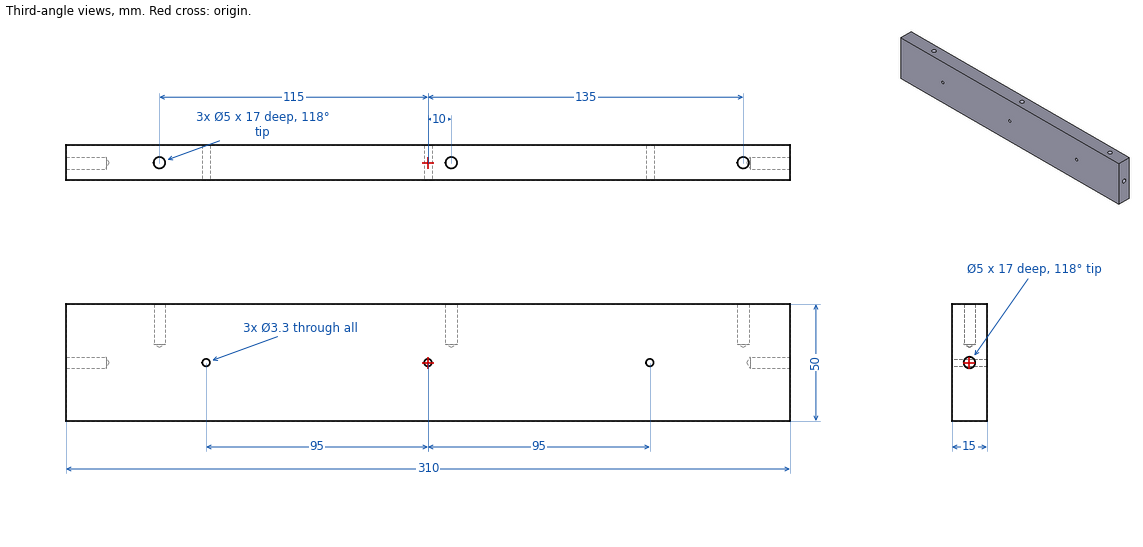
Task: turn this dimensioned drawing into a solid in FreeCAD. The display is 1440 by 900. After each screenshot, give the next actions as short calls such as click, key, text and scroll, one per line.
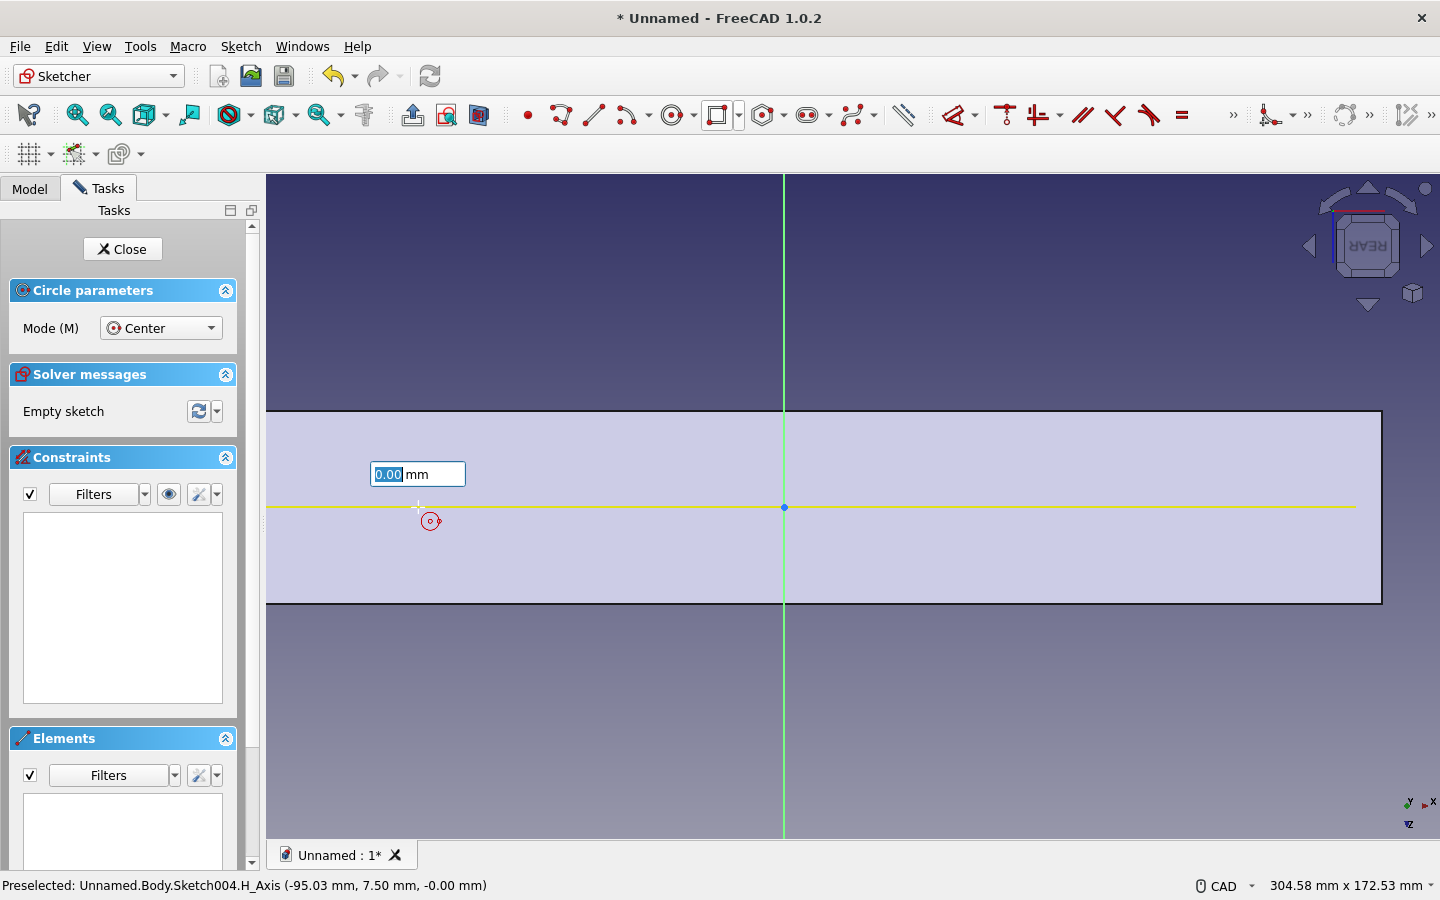
scroll(416, 513, up, 5)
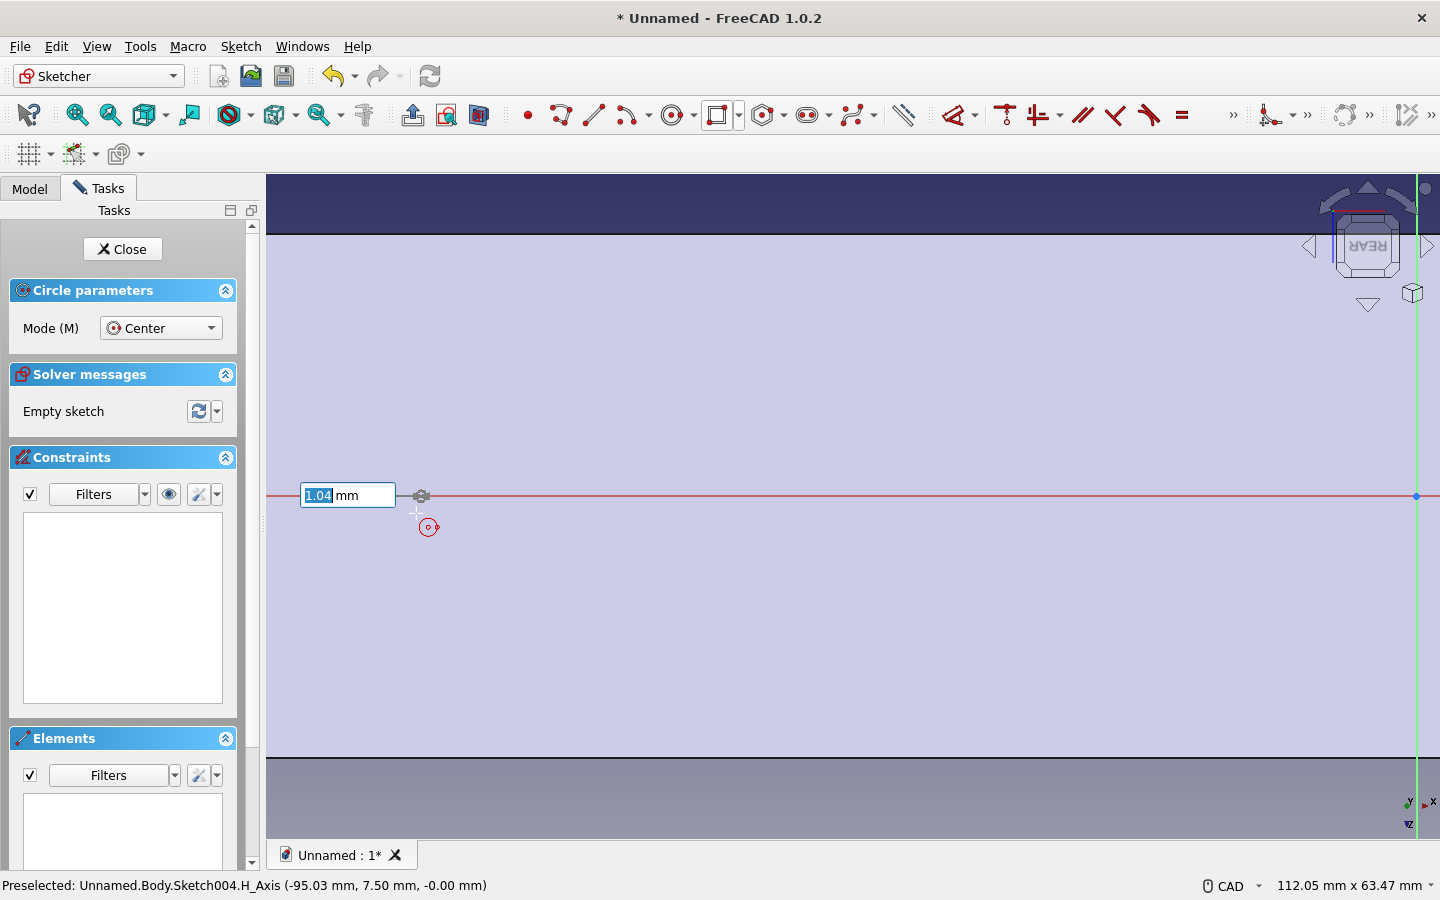
click(416, 513)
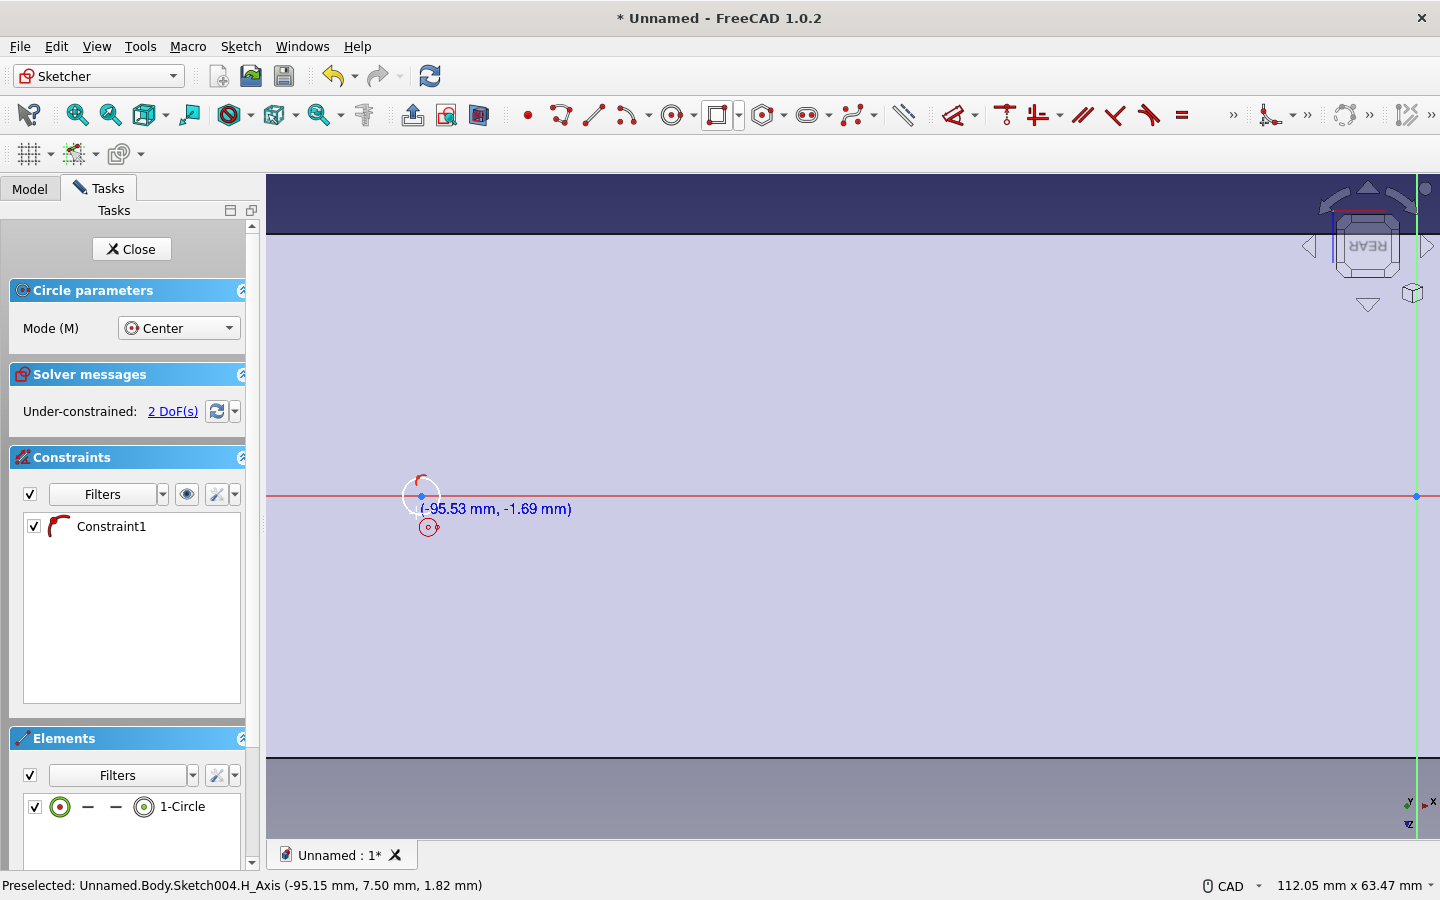
scroll(416, 512, down, 5)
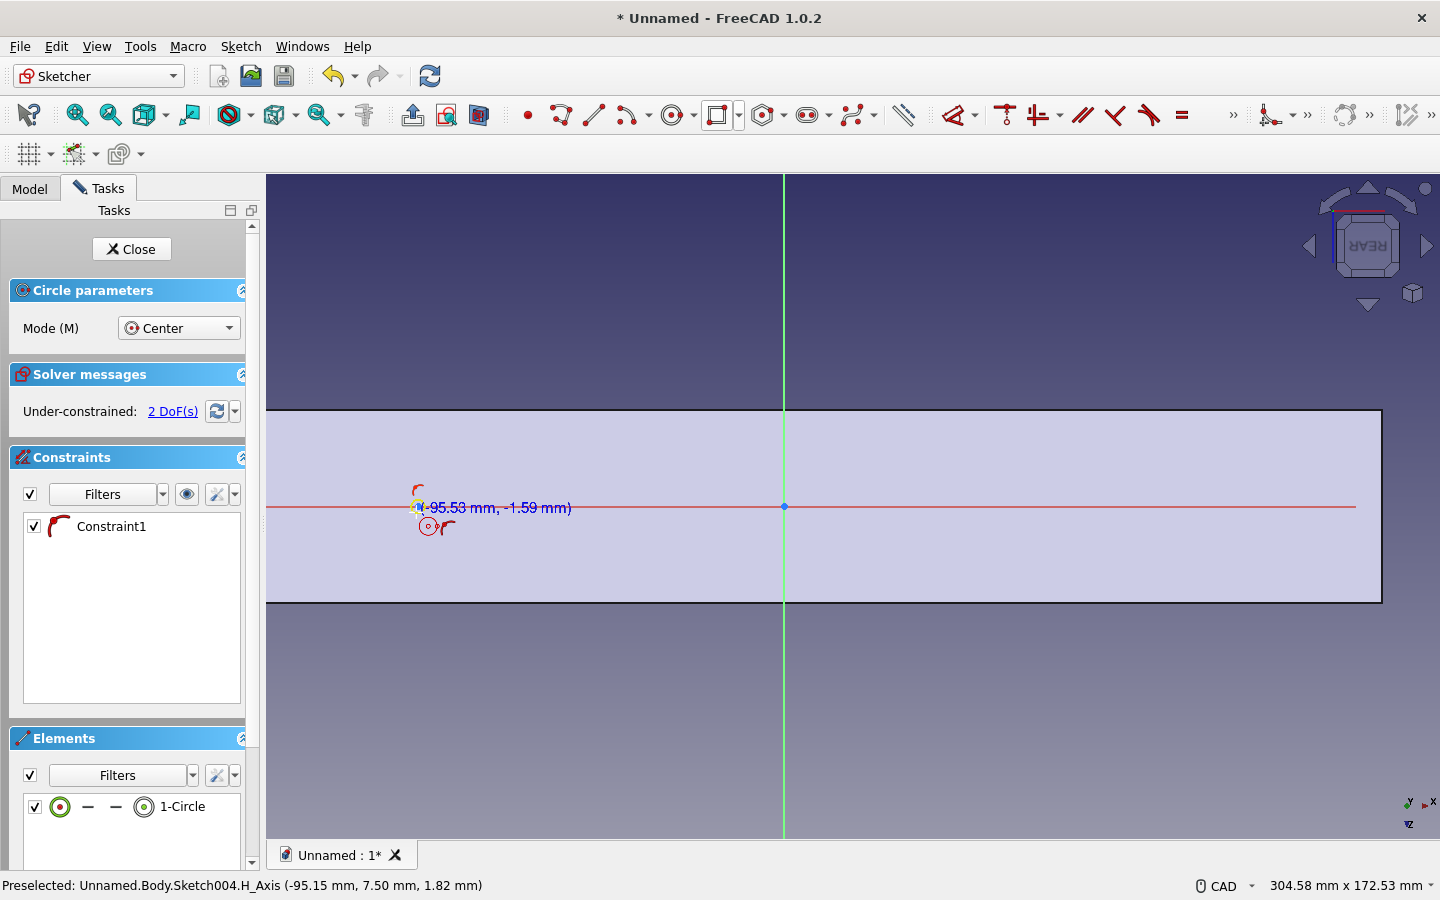
scroll(784, 507, up, 7)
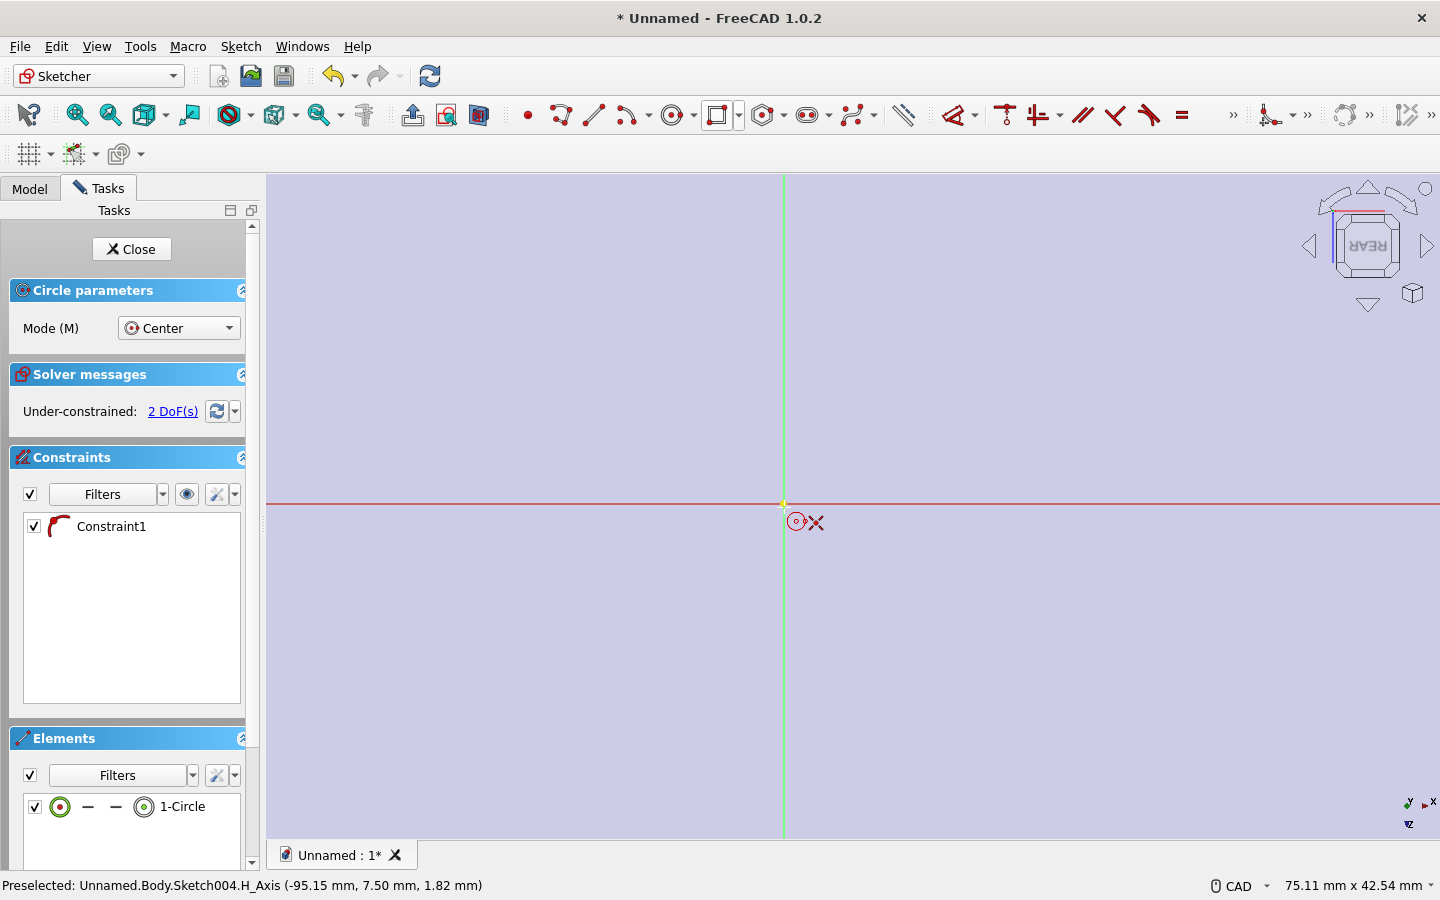
scroll(785, 507, down, 7)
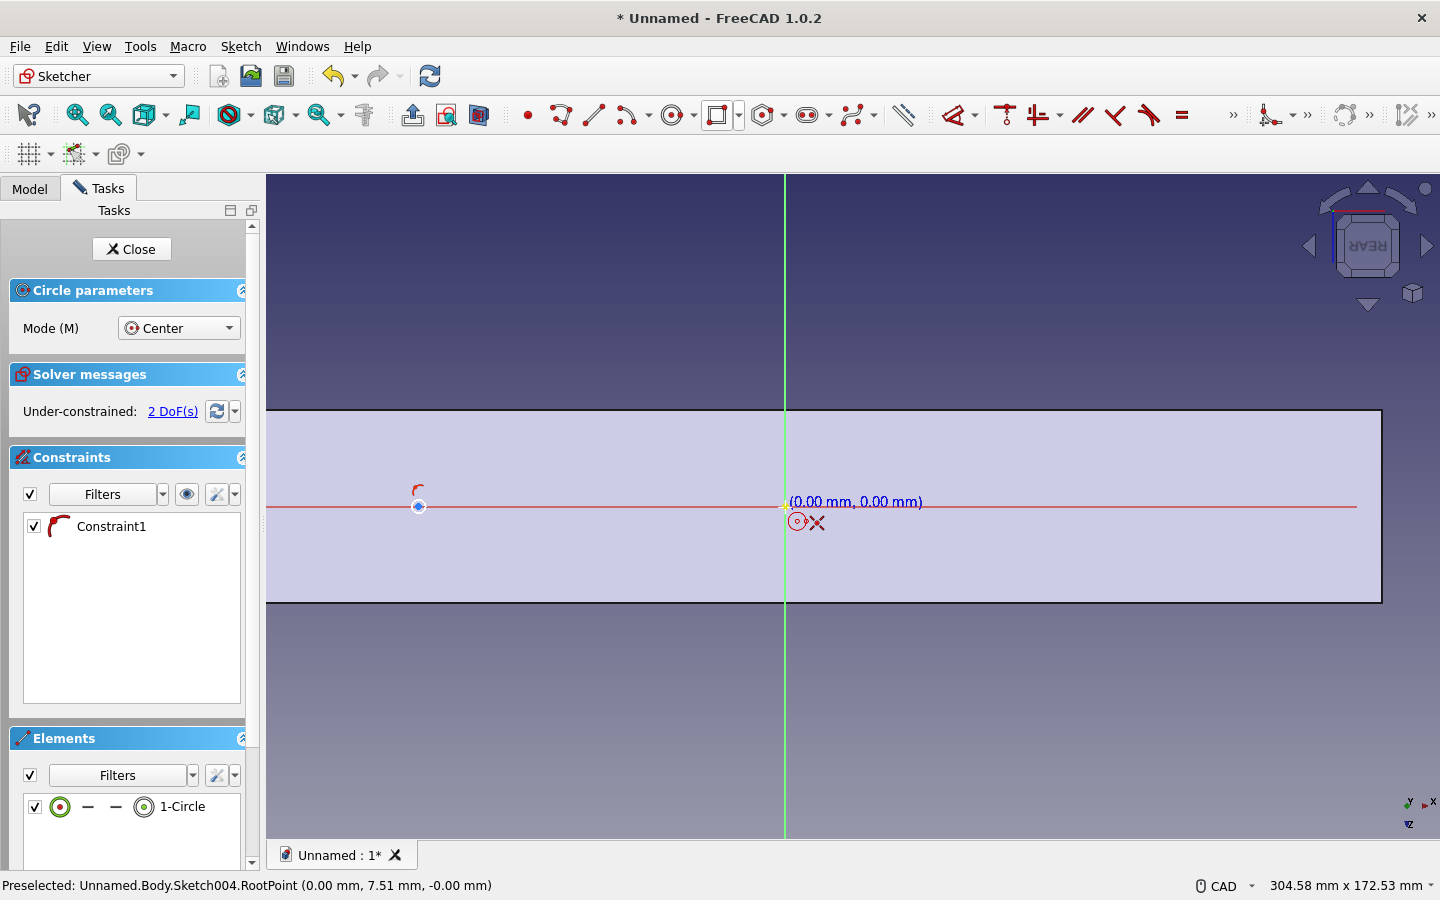
click(785, 507)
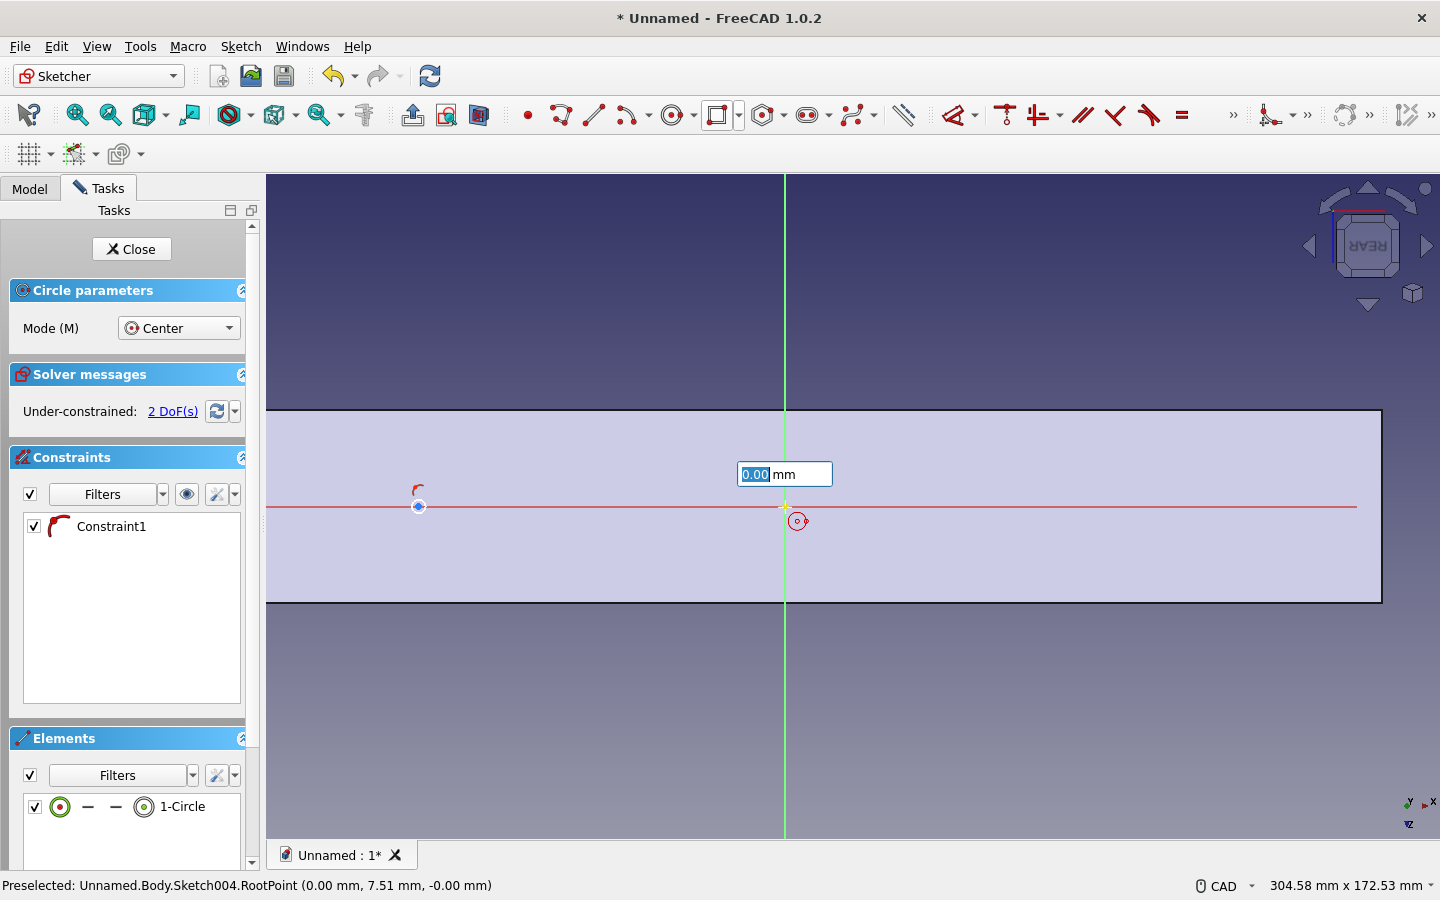
scroll(790, 502, up, 7)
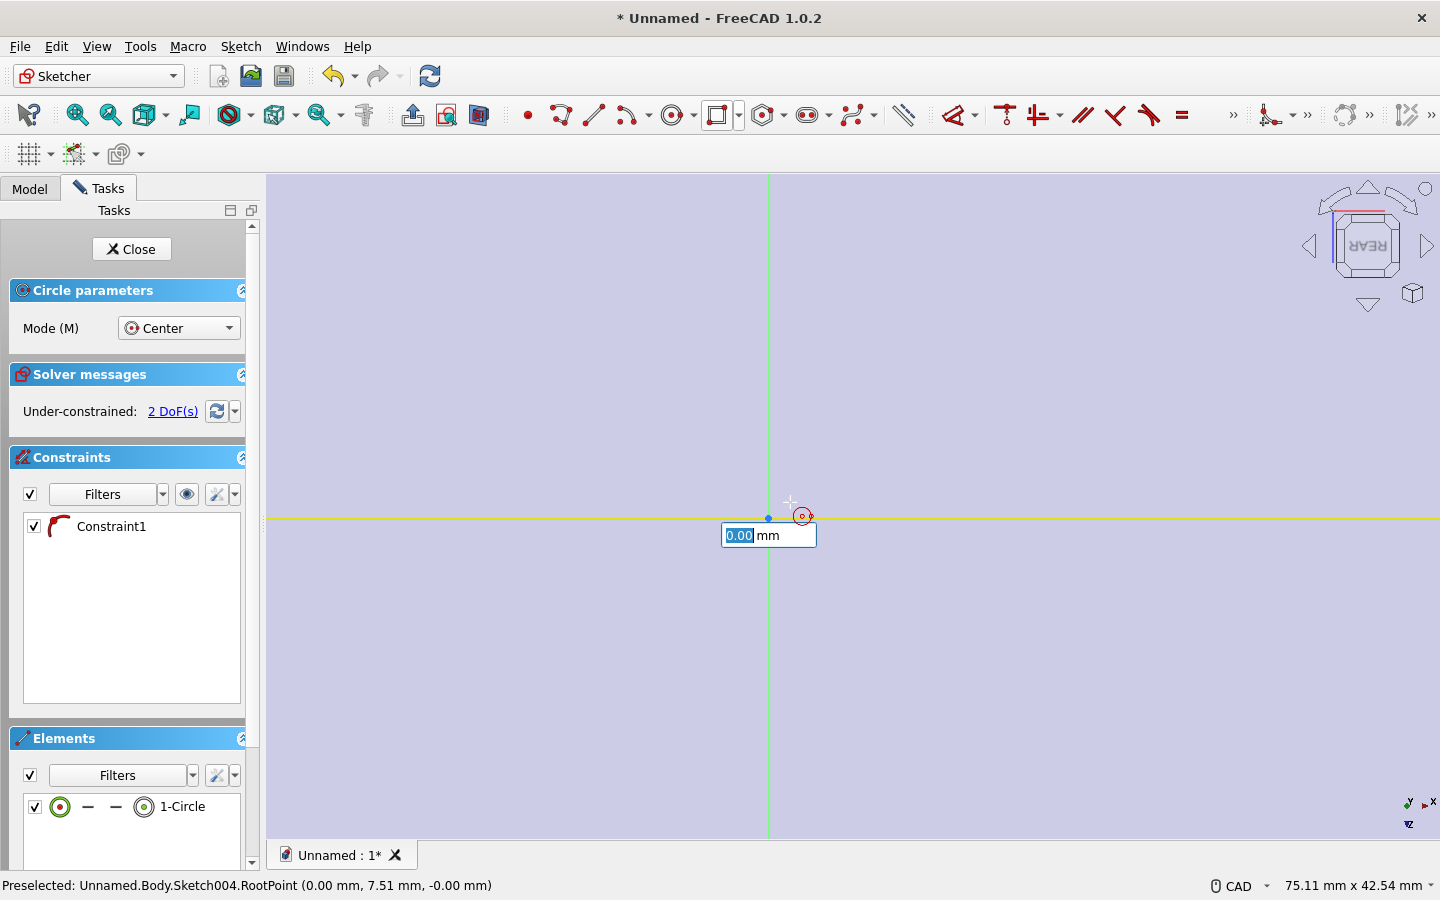
click(787, 501)